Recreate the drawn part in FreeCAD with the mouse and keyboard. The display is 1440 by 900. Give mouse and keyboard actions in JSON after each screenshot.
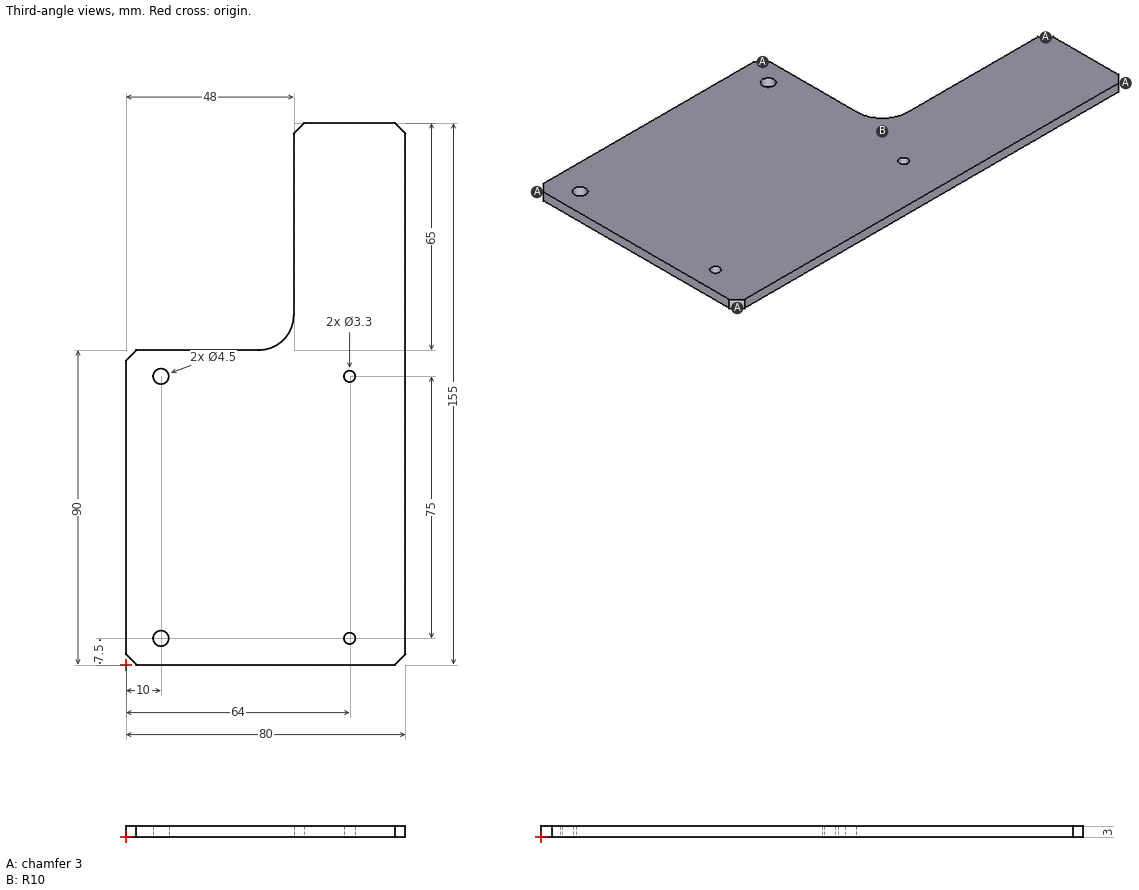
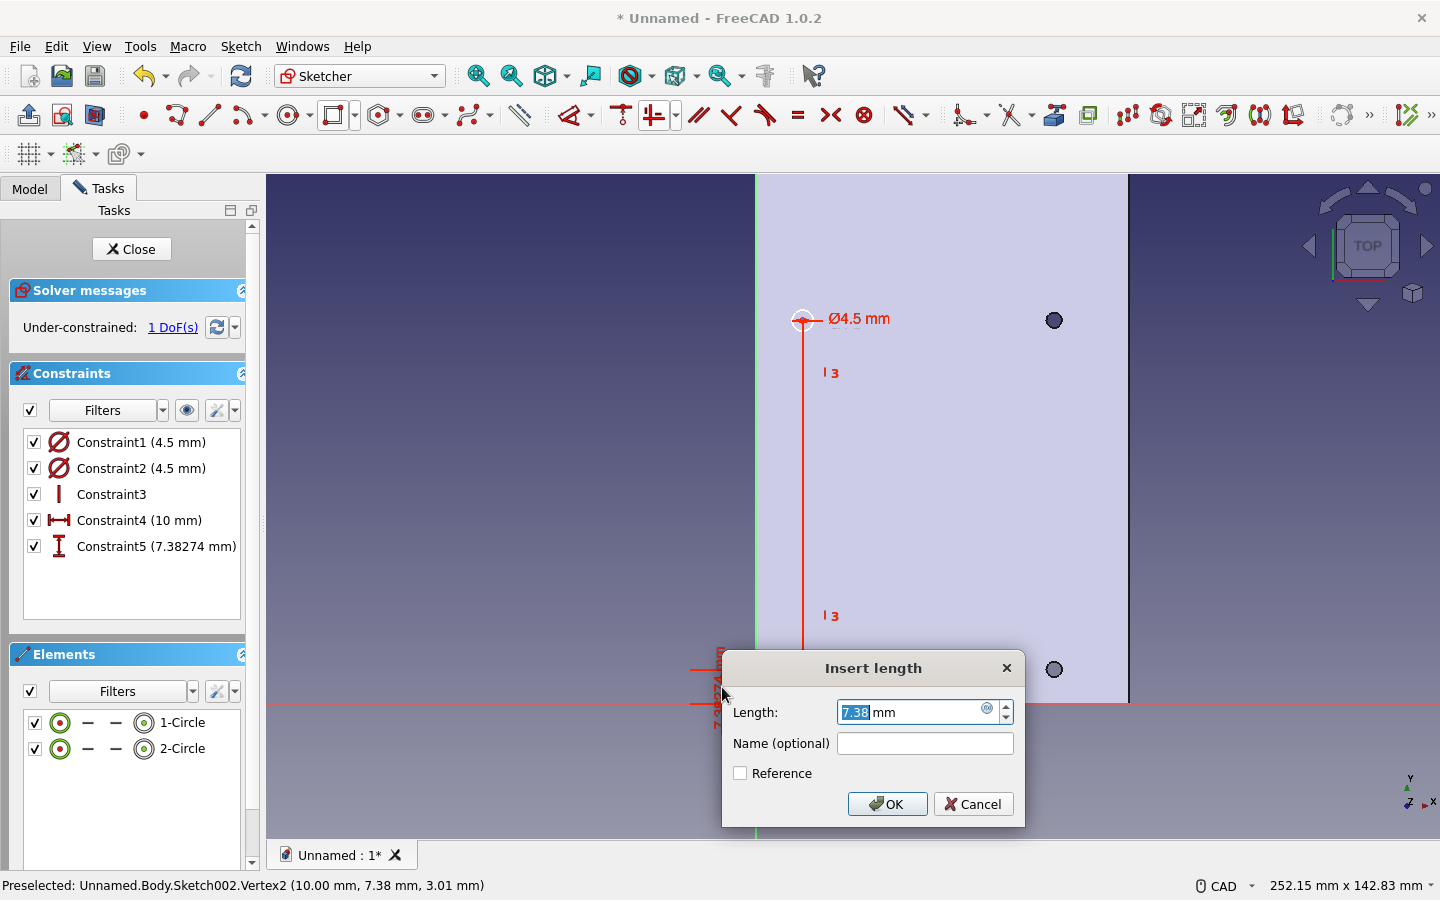
{"action": "type", "text": "7.5"}
{"action": "key", "text": "Return"}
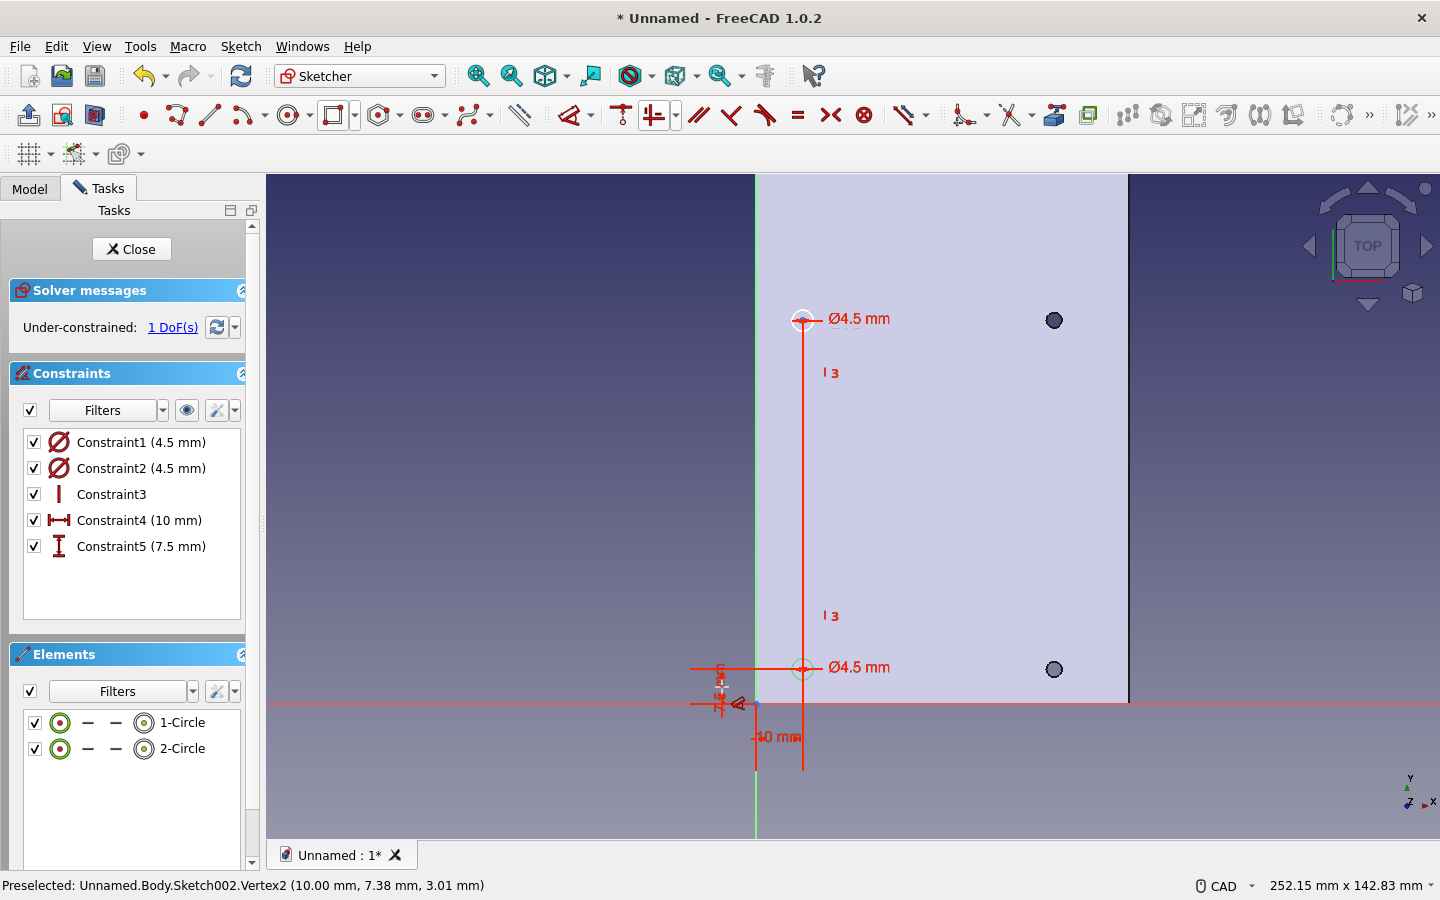
{"action": "left_click", "coordinate": [803, 321]}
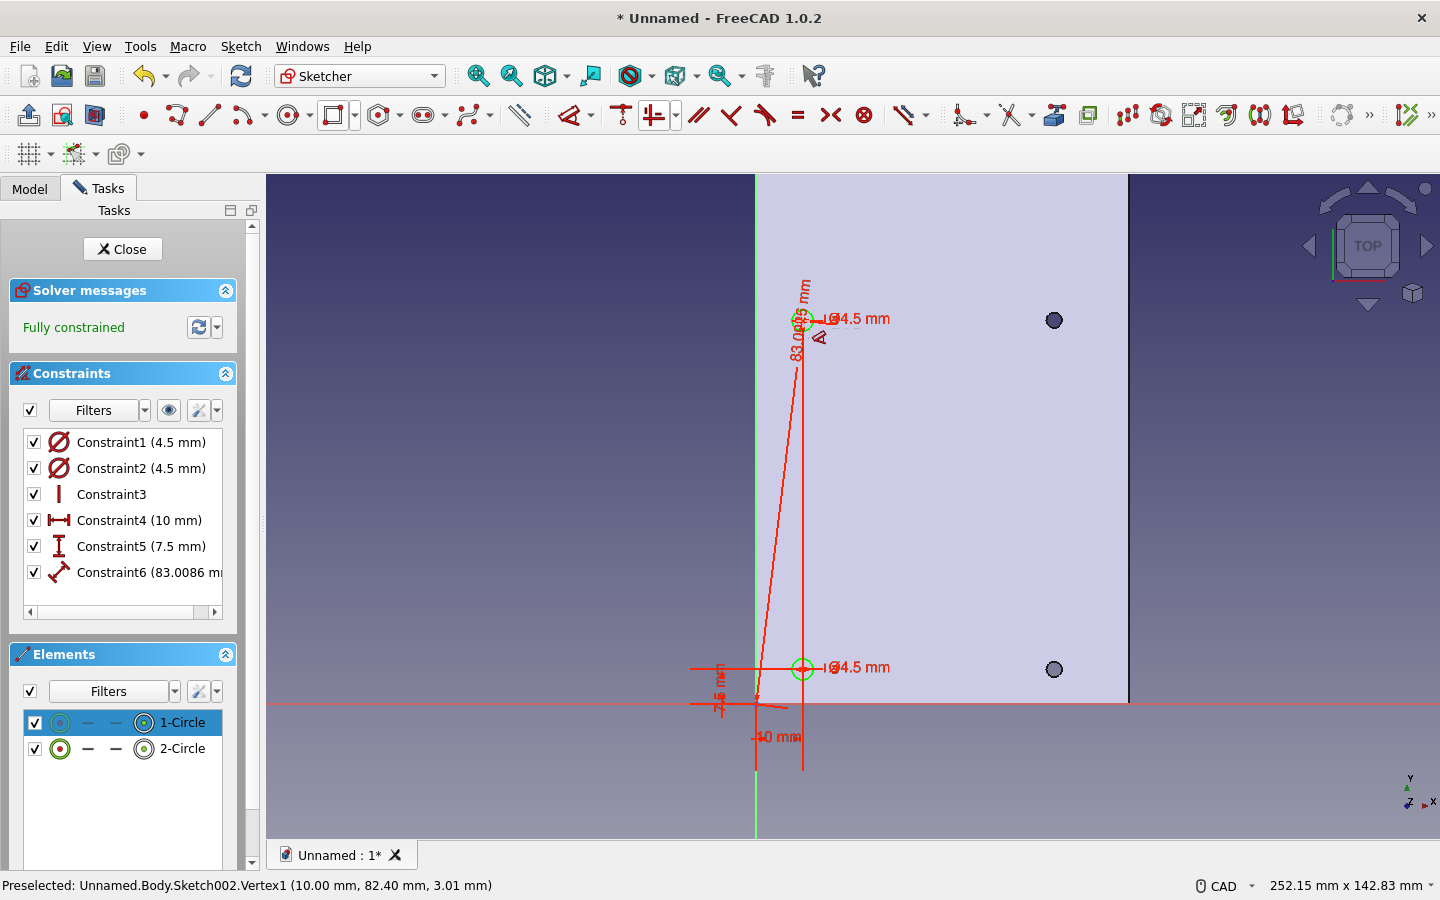
{"action": "left_click", "coordinate": [803, 669]}
{"action": "left_click", "coordinate": [837, 495]}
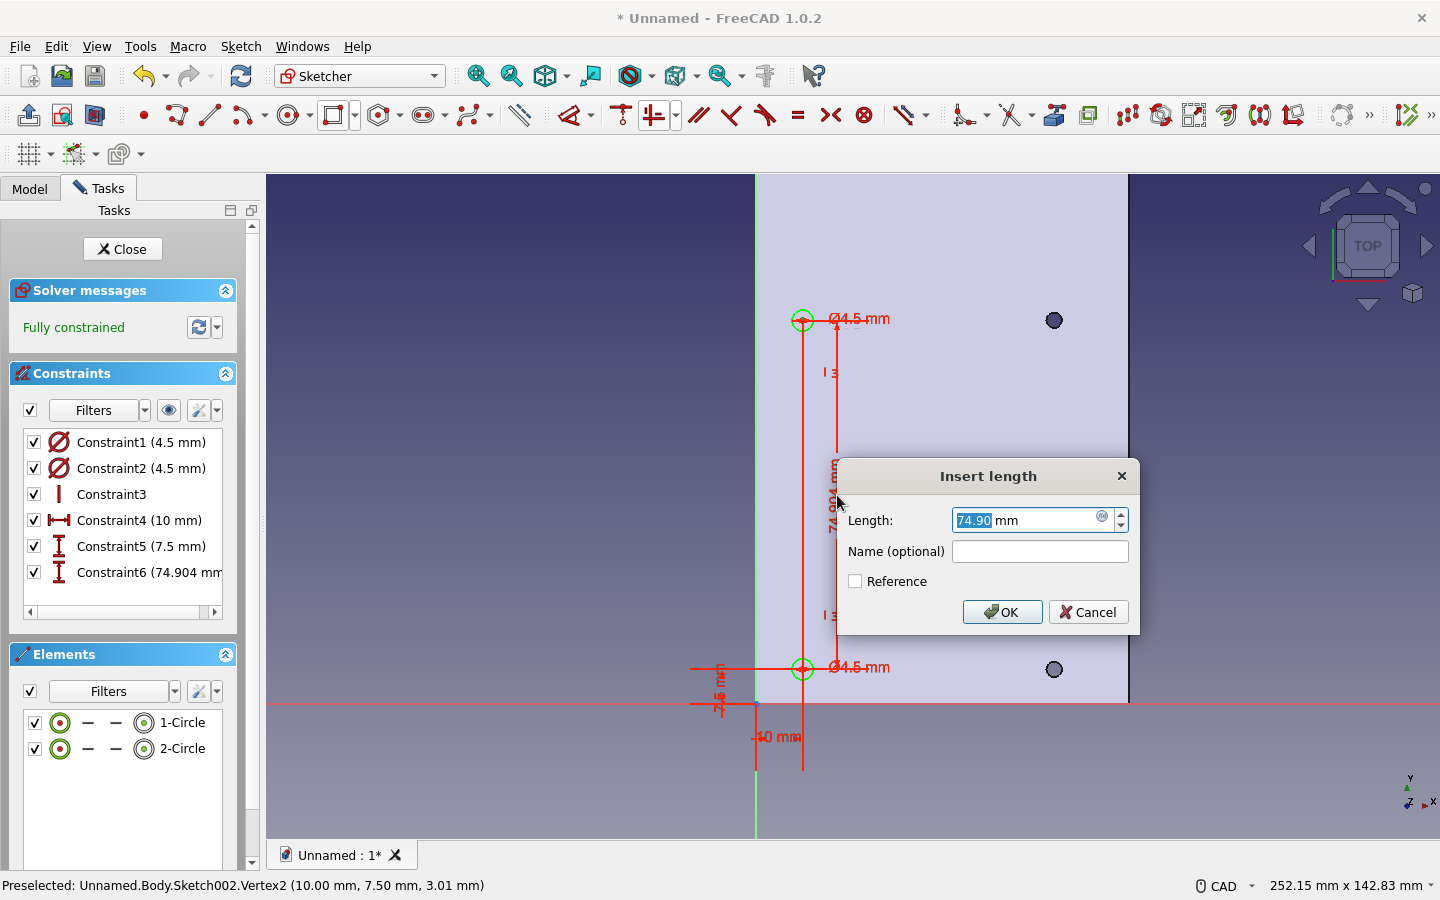
{"action": "type", "text": "75"}
{"action": "key", "text": "Return"}
{"action": "key", "text": "Escape"}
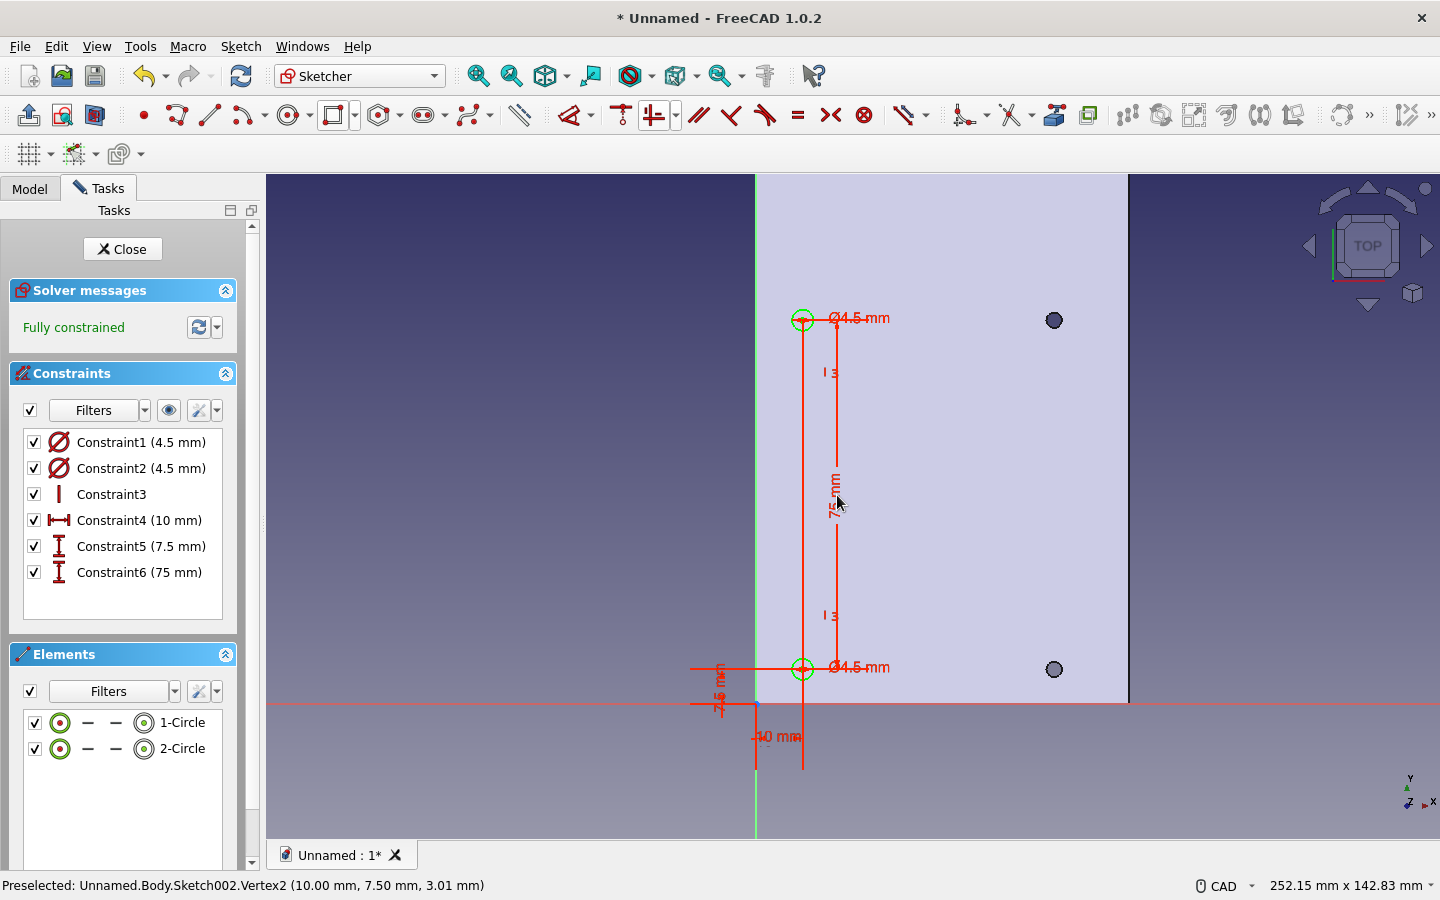
{"action": "left_click", "coordinate": [123, 249]}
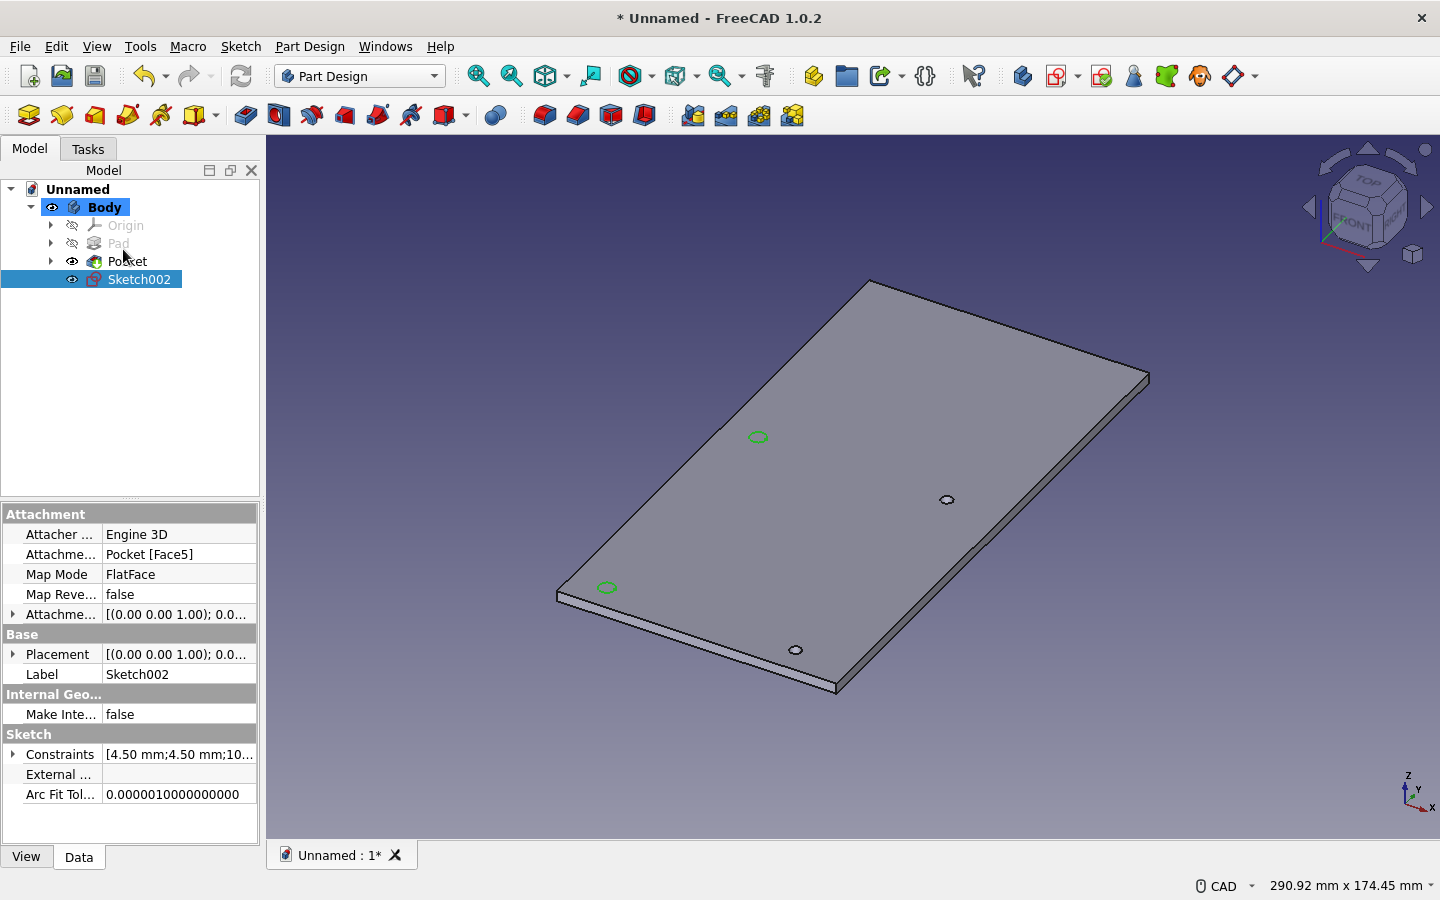
{"action": "left_click", "coordinate": [246, 116]}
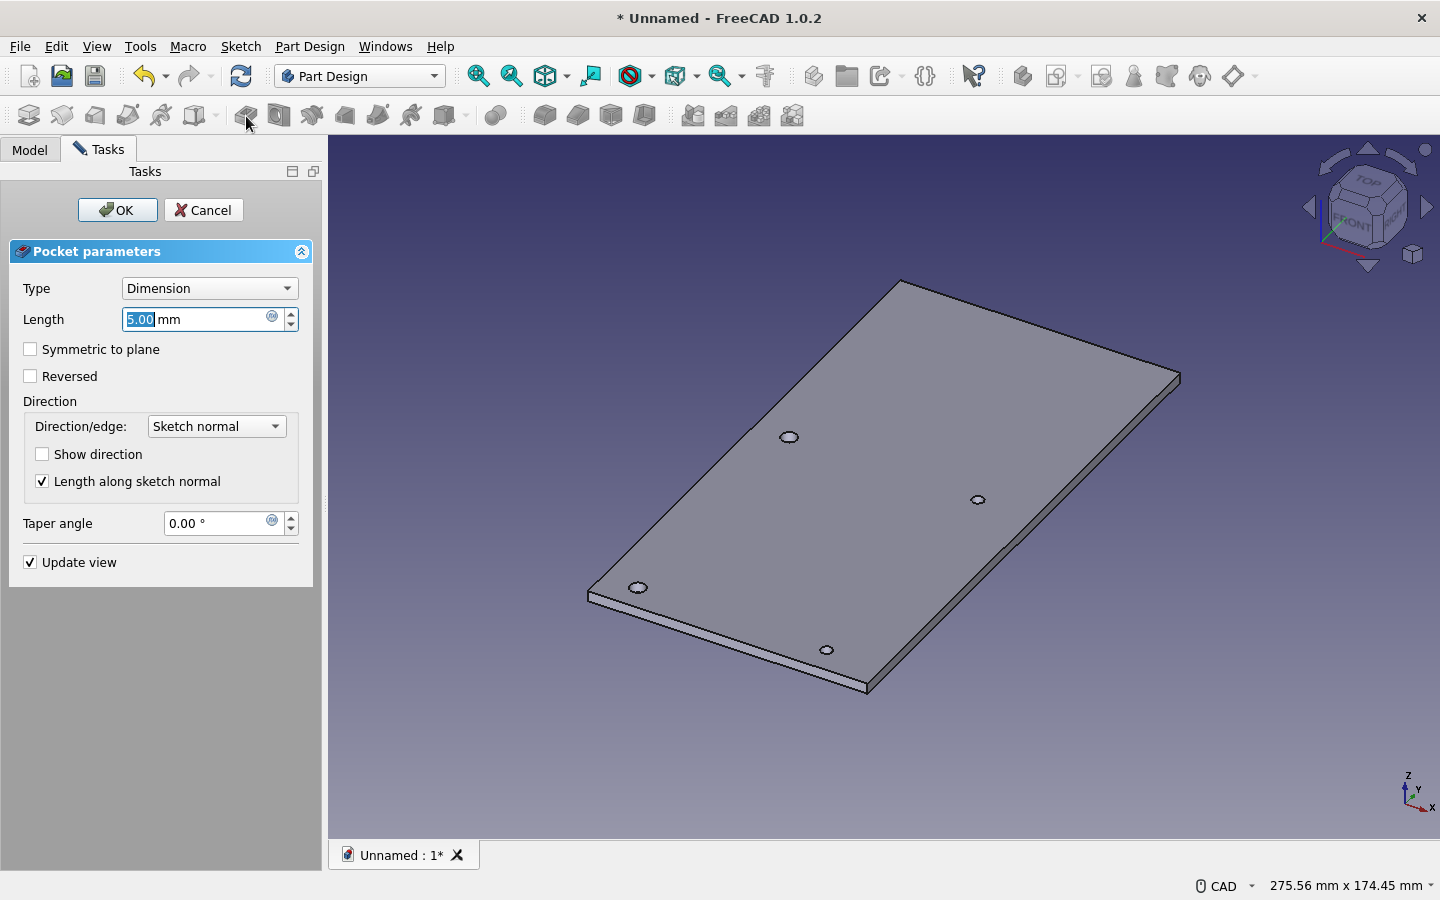
{"action": "left_click", "coordinate": [210, 288]}